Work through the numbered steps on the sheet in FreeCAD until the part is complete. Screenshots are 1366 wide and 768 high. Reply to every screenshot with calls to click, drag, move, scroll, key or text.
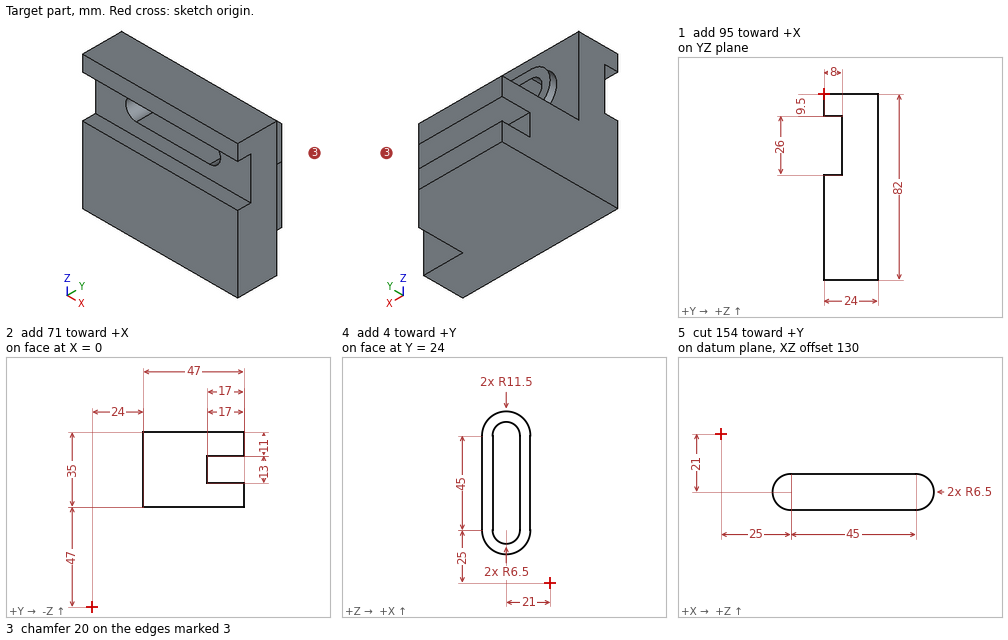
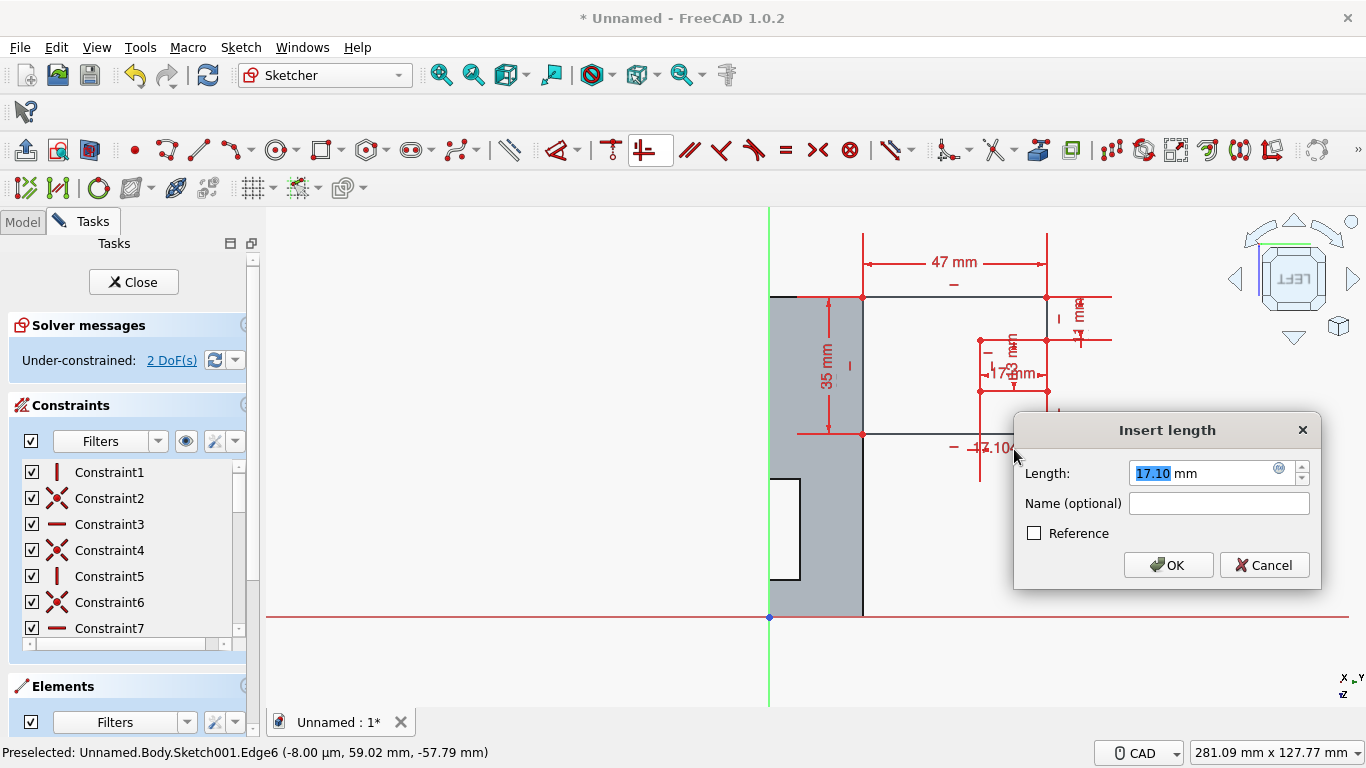
text(17)
key(Return)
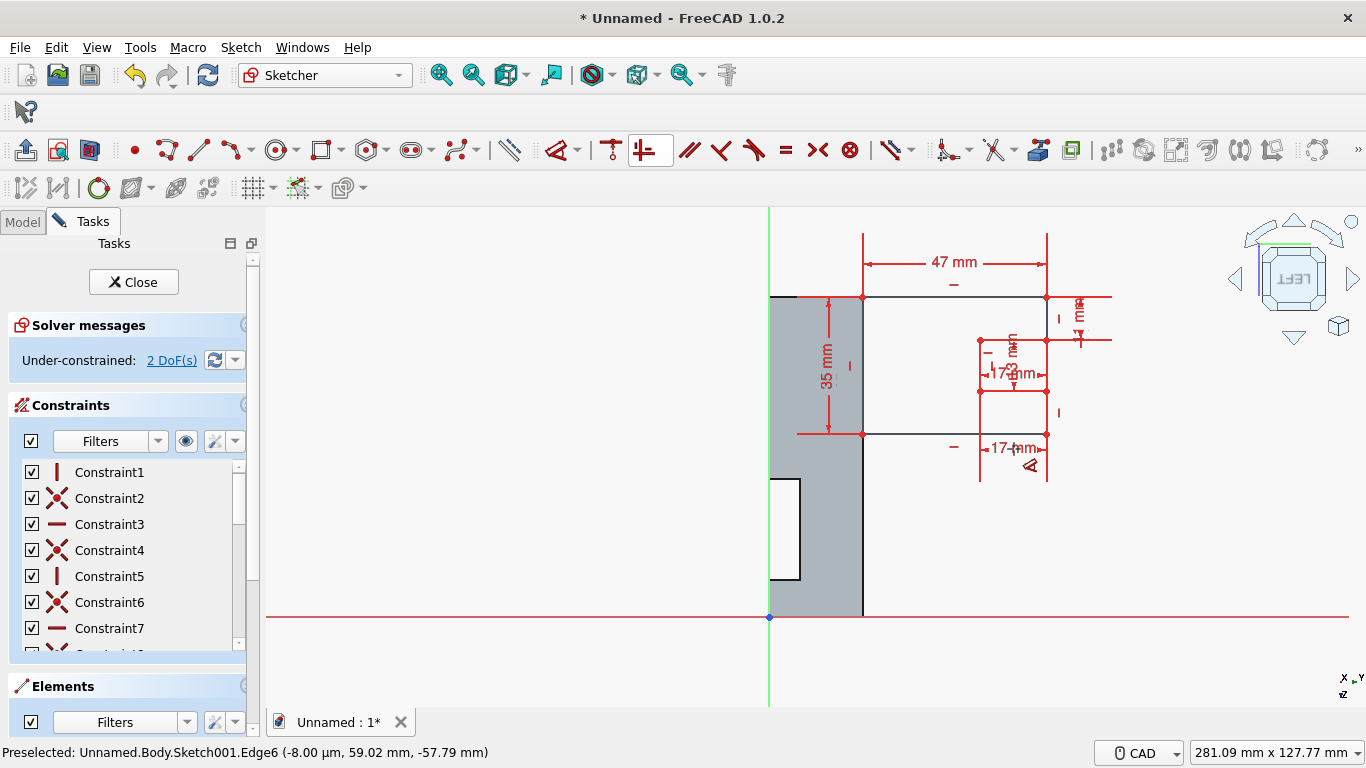
click(863, 434)
click(816, 651)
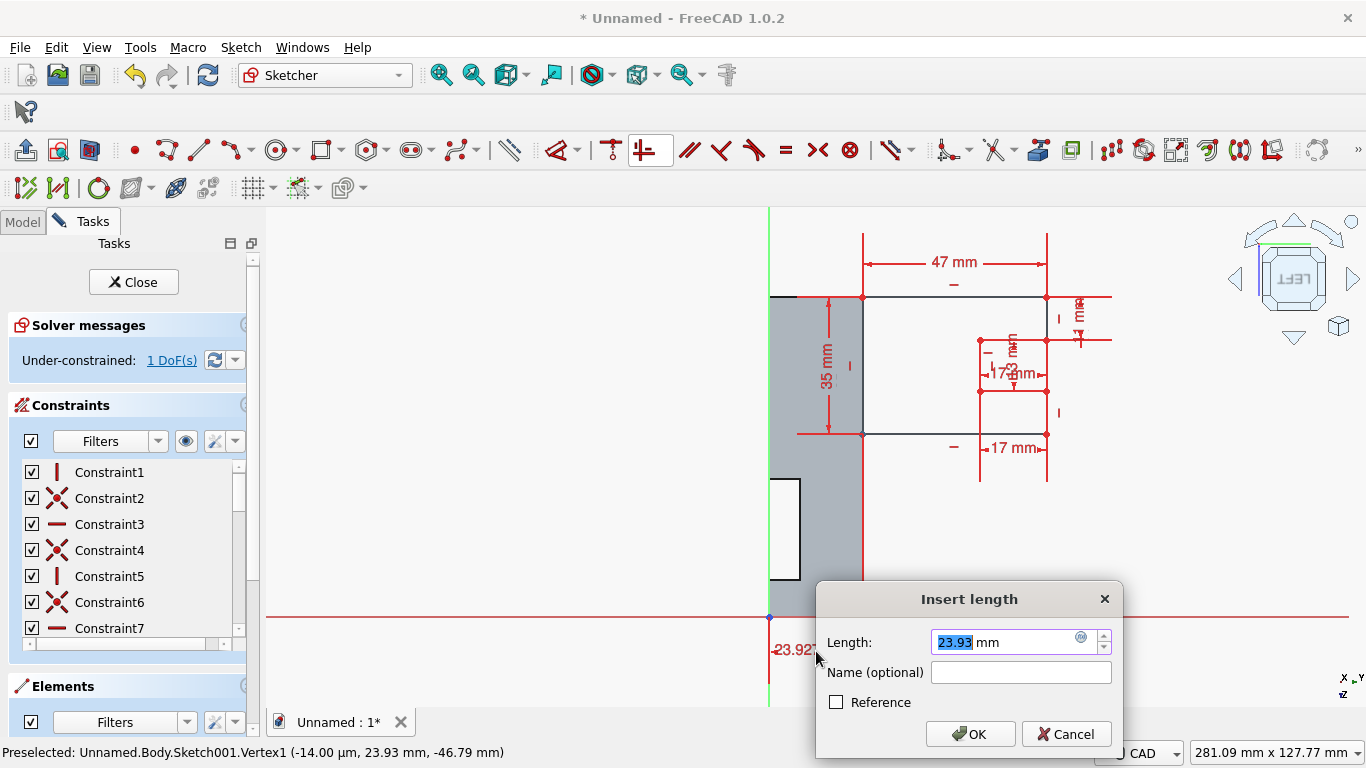
text(24)
key(Return)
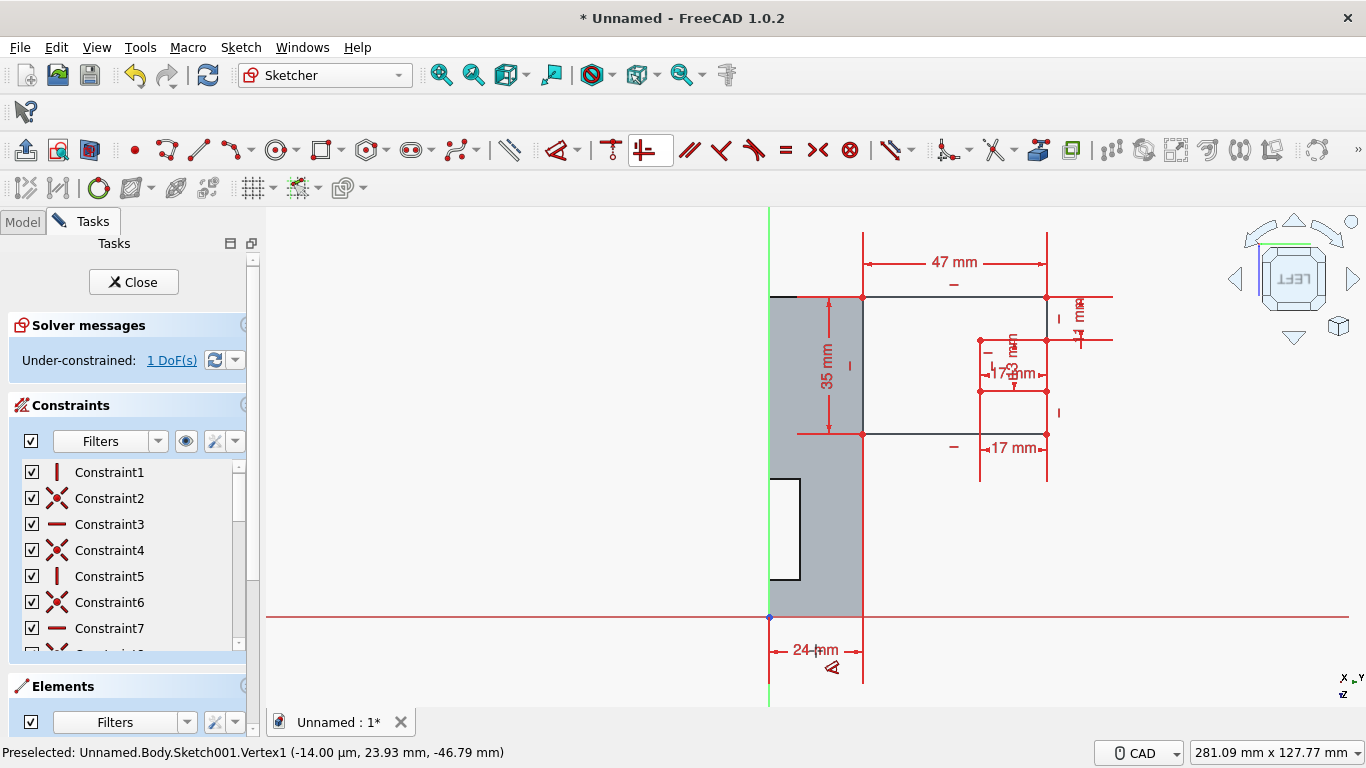
click(863, 434)
click(735, 526)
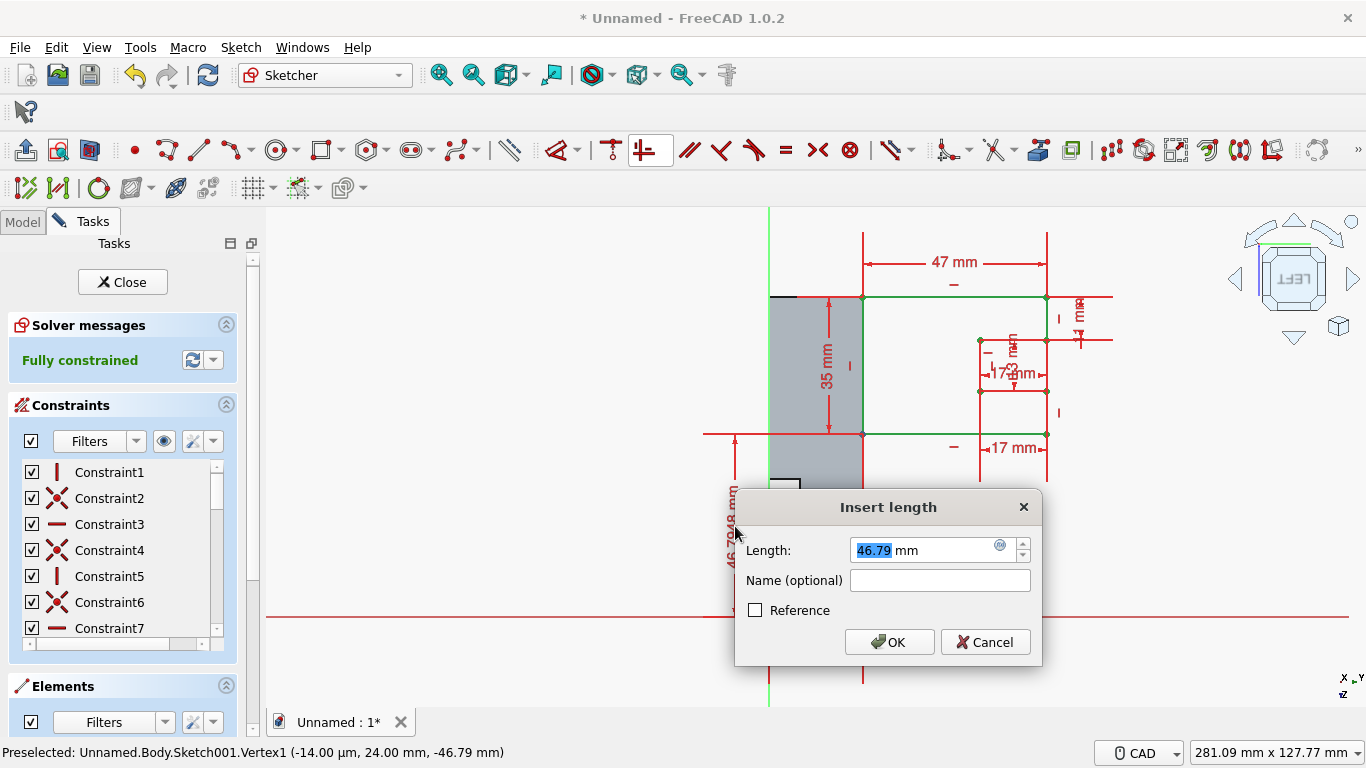
text(47)
key(Return)
key(Escape)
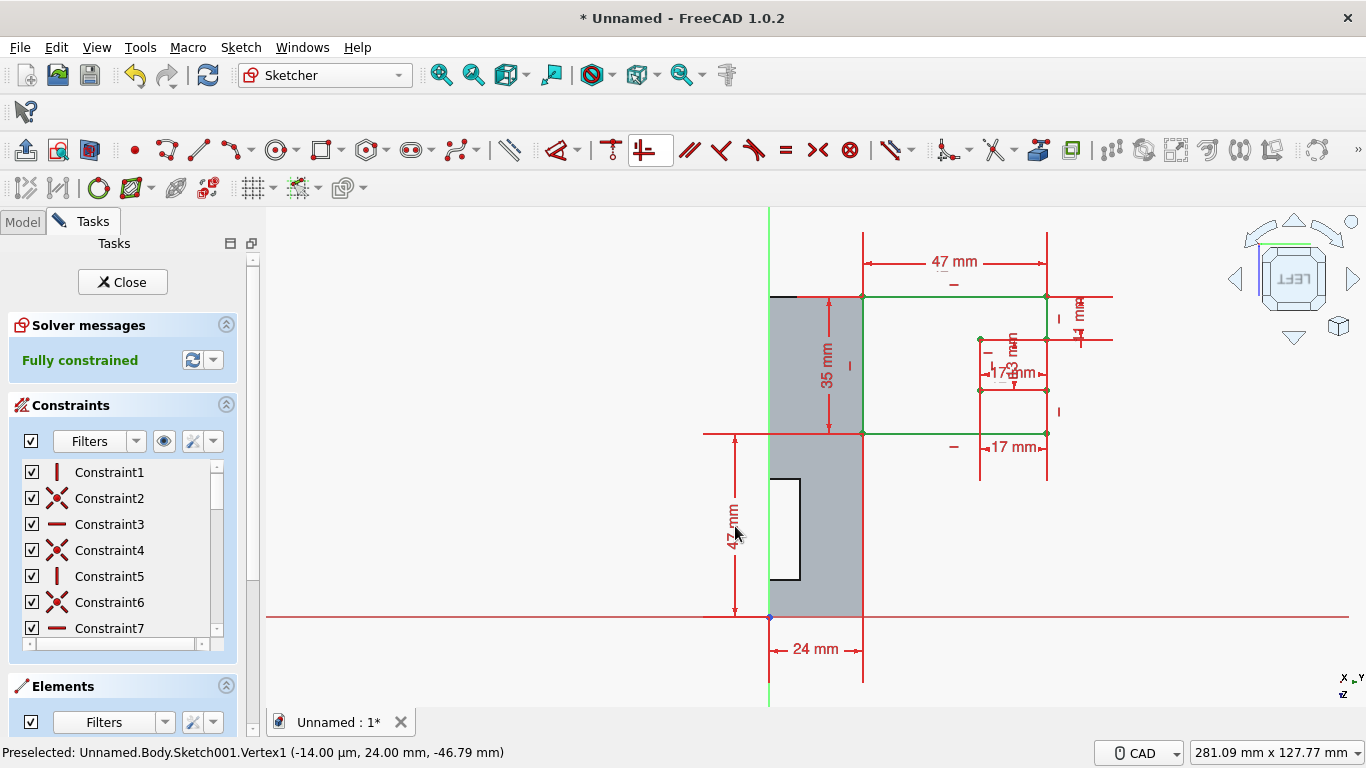
click(123, 282)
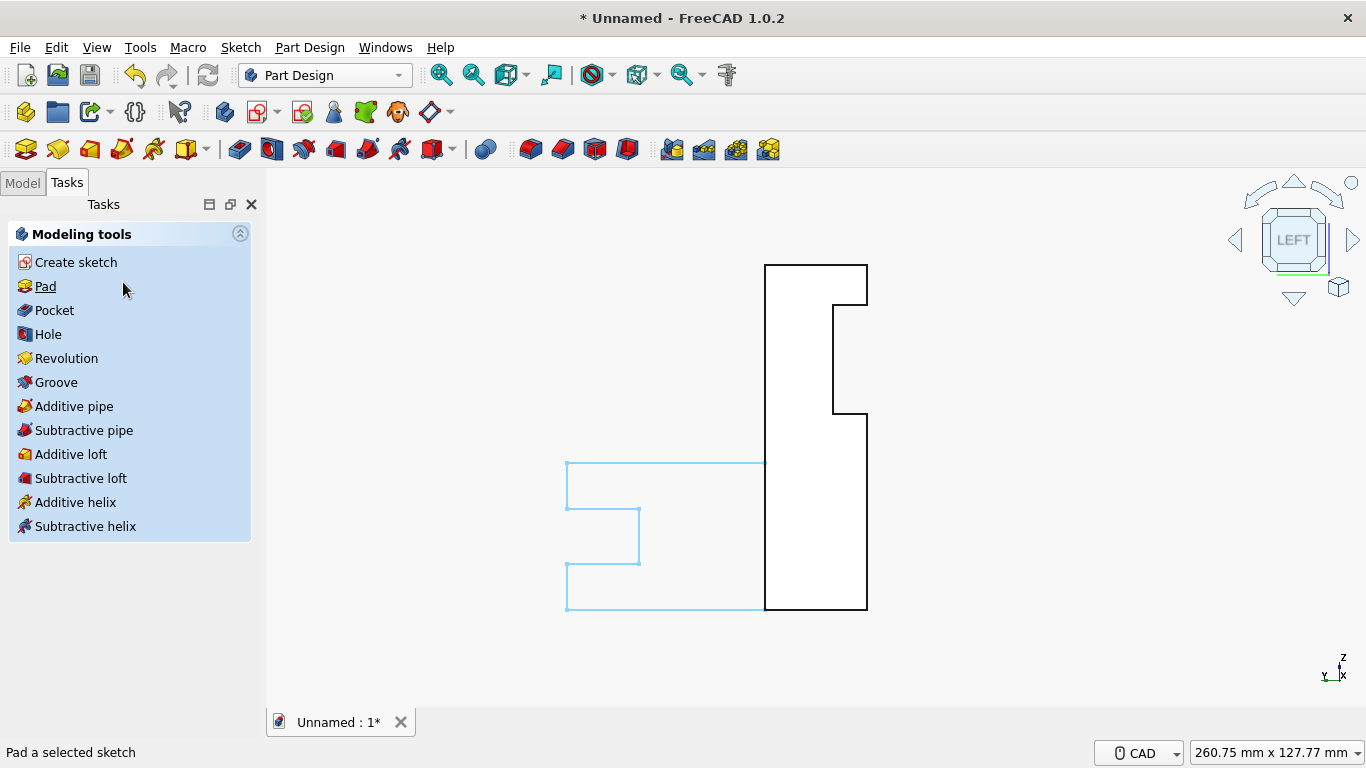
click(26, 150)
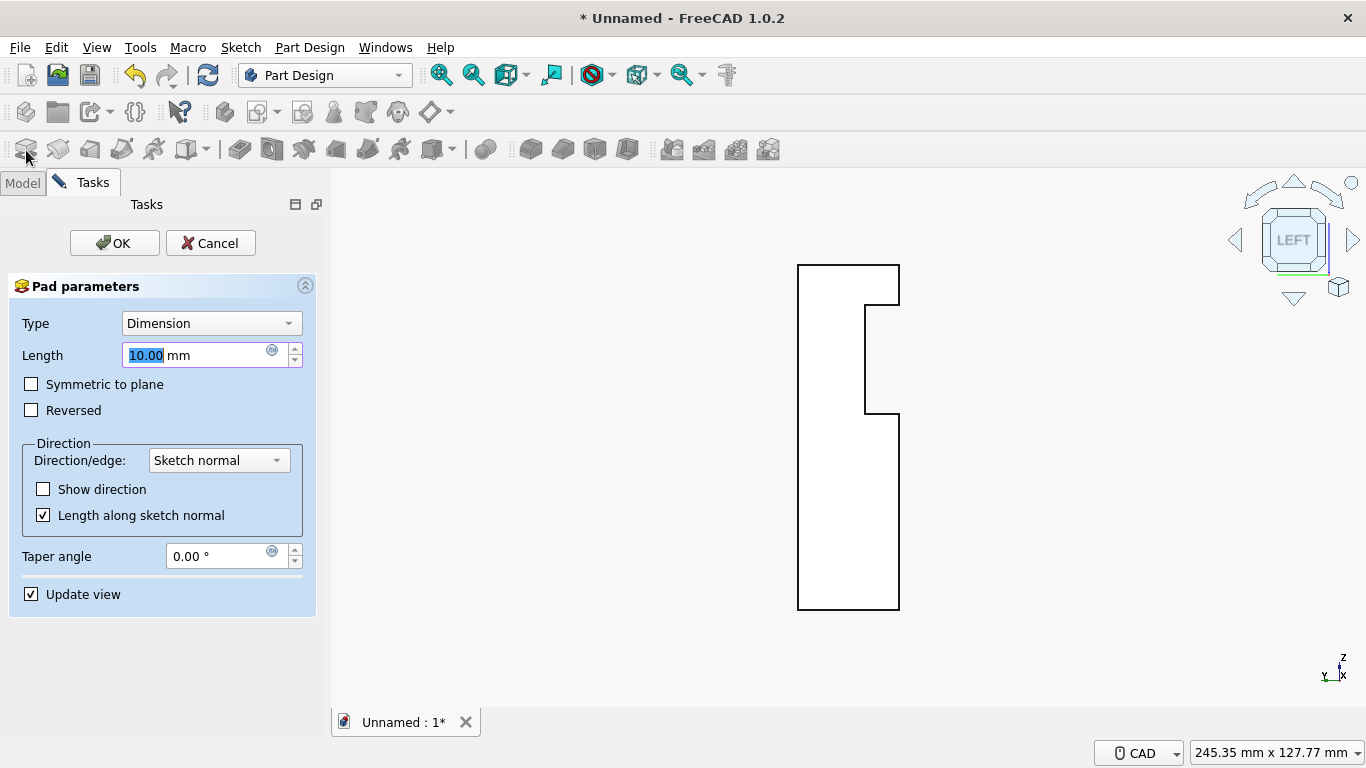
text(71)
key(Tab)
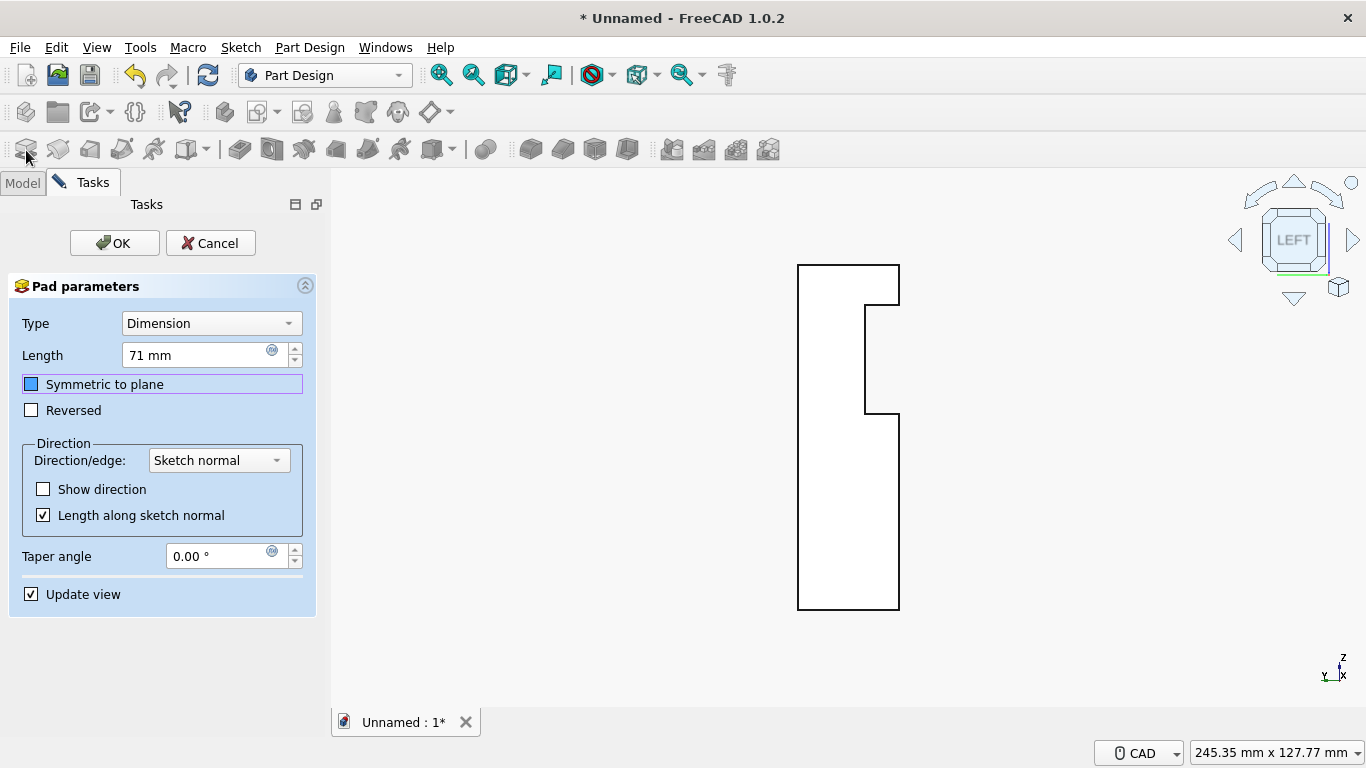
click(30, 410)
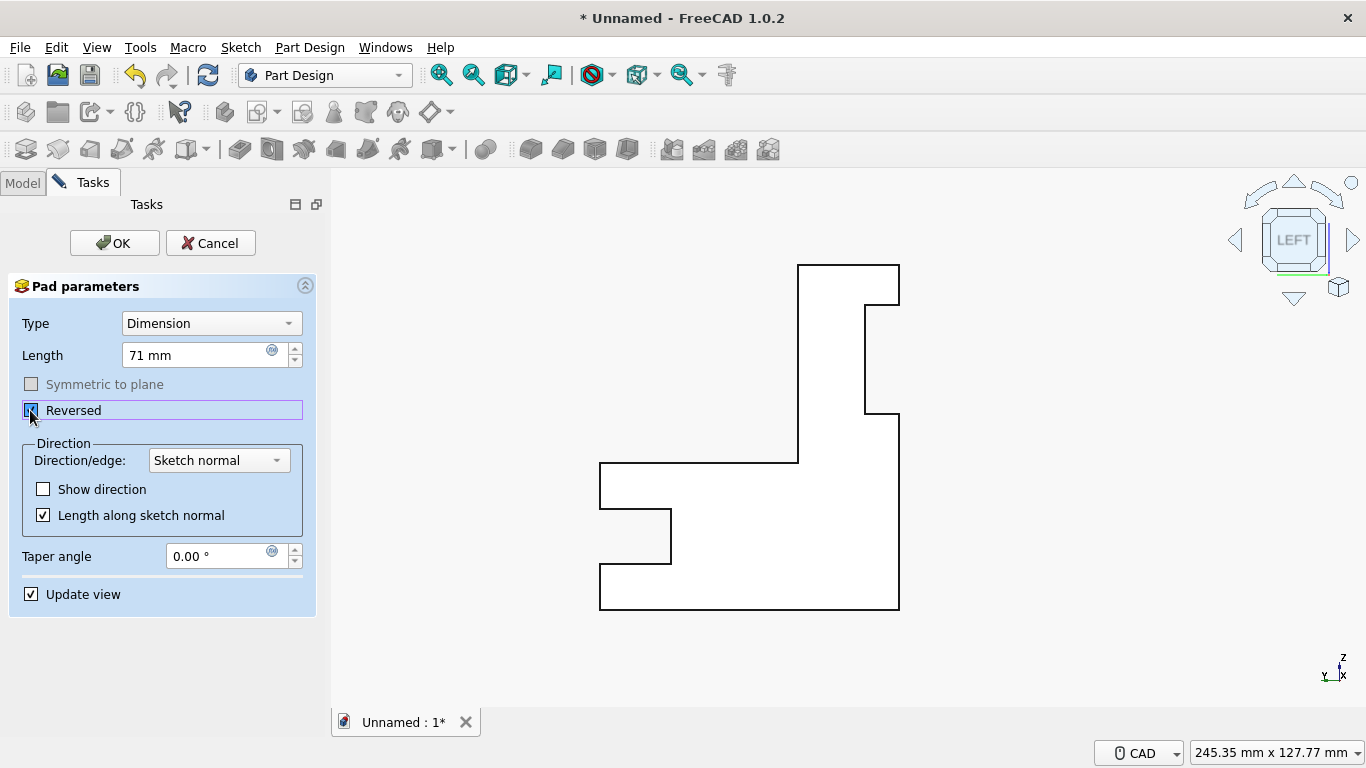
click(115, 243)